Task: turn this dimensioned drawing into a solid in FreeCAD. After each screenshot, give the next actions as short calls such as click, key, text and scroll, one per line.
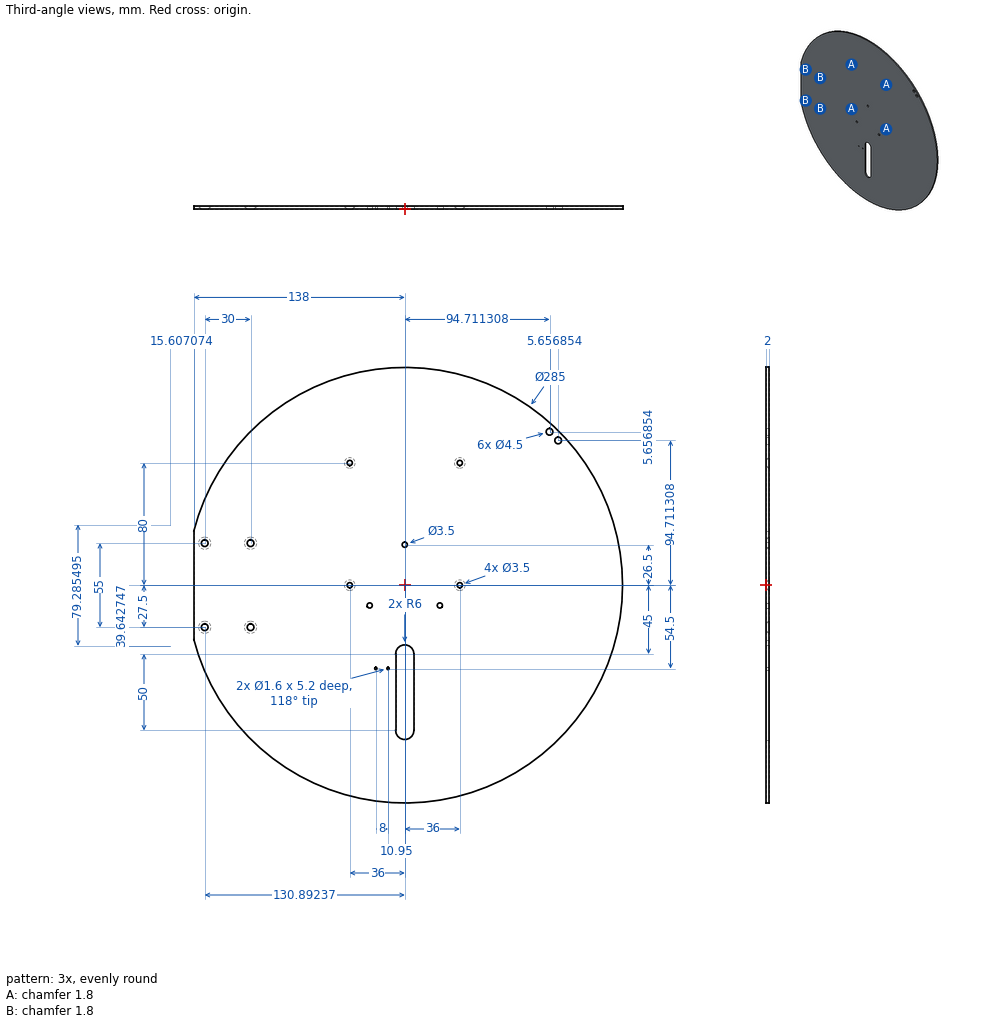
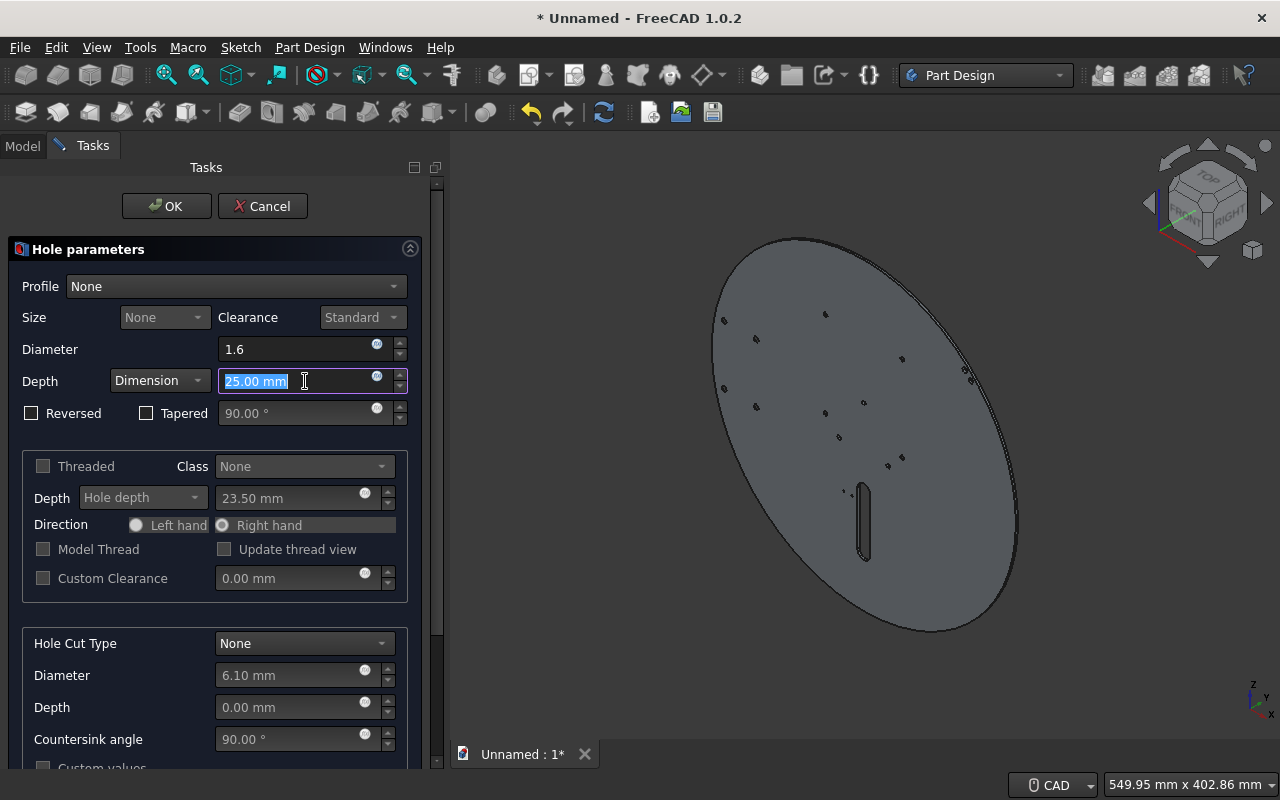
text(5.2)
key(Tab)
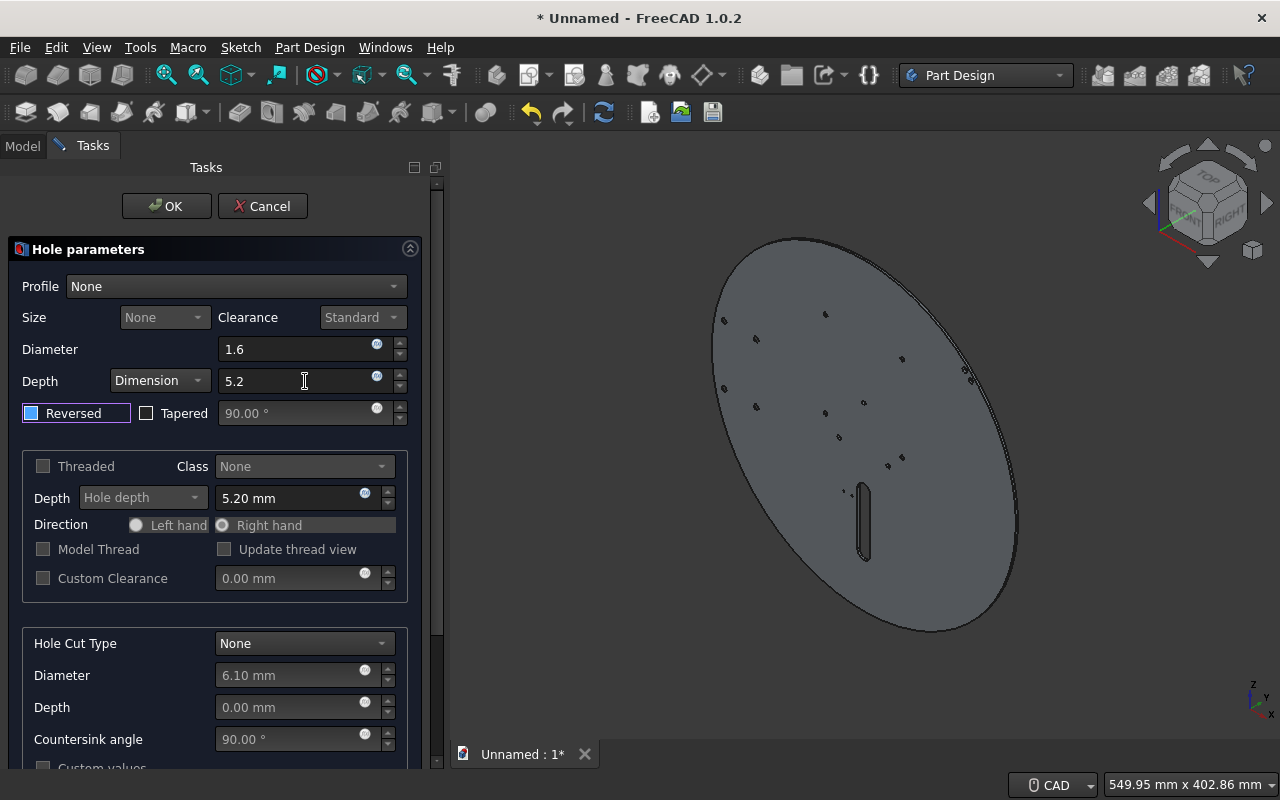
click(167, 206)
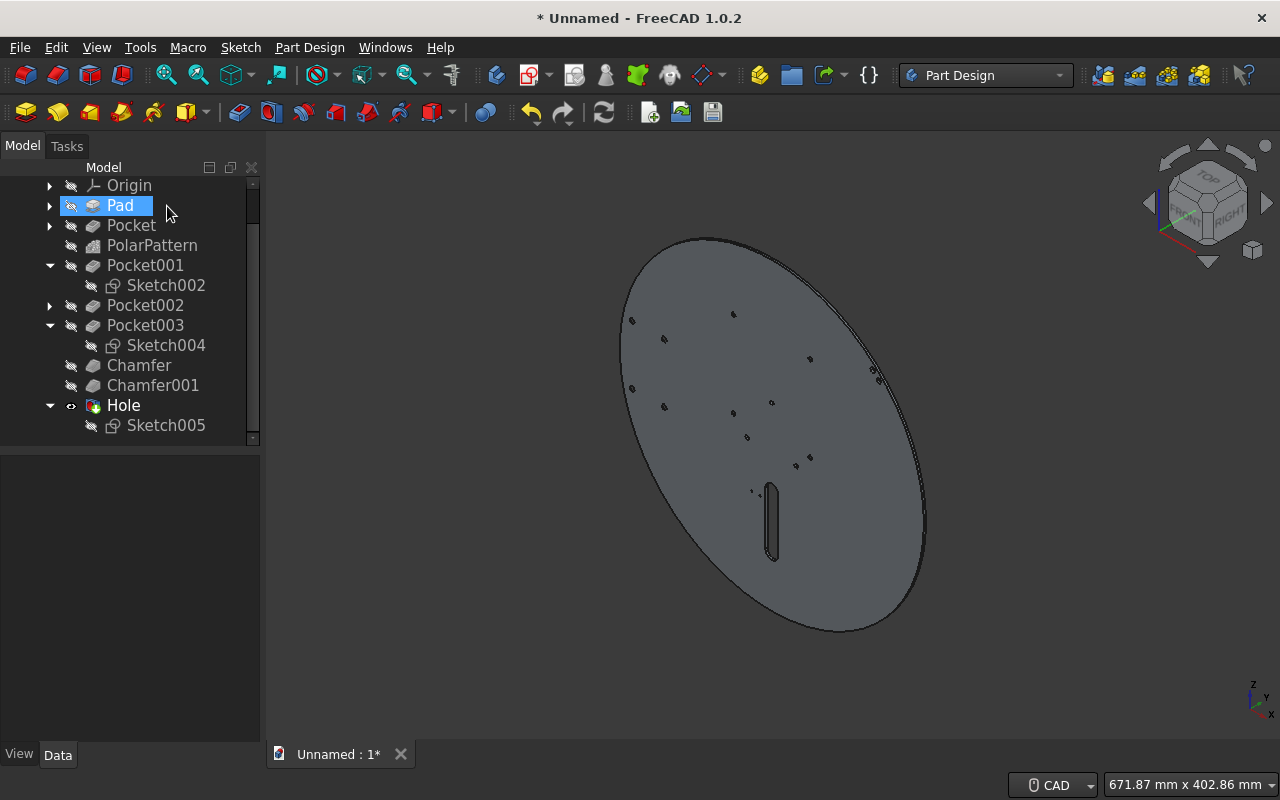
key(4)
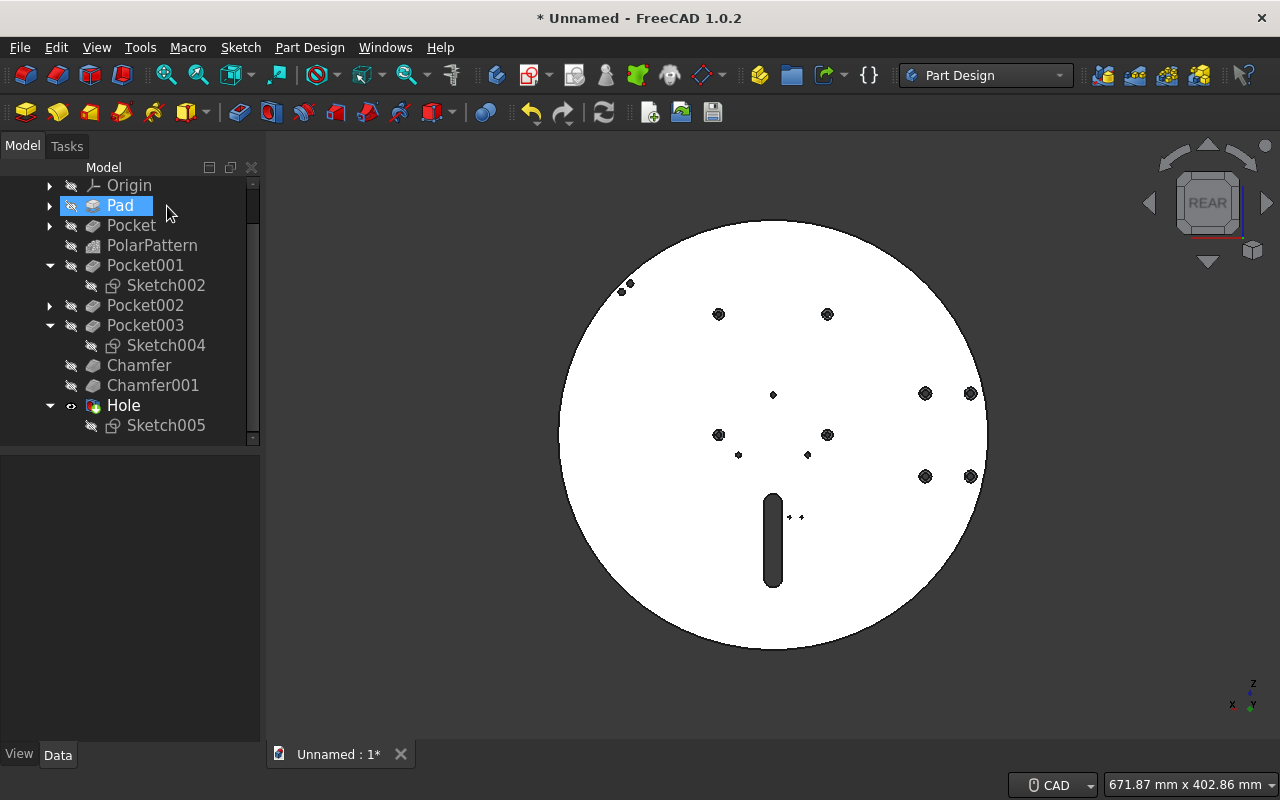
click(650, 495)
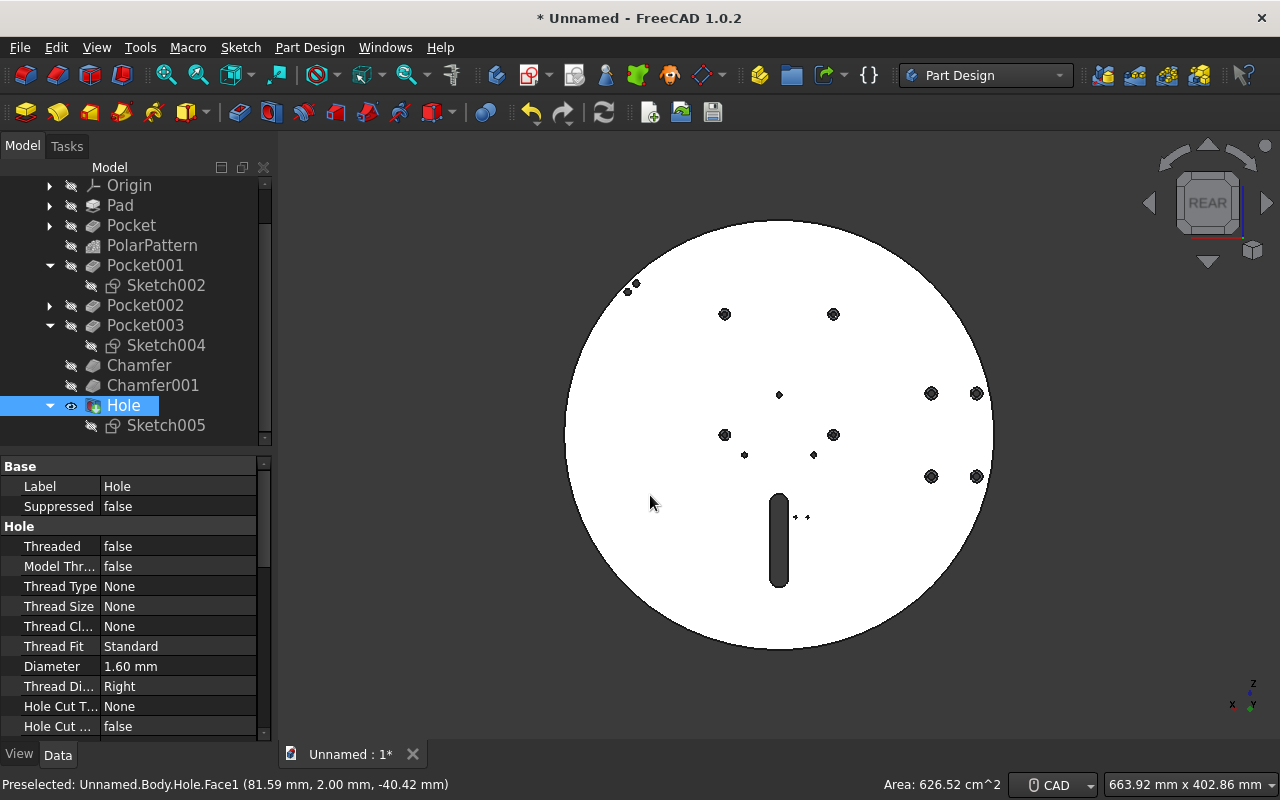
click(530, 76)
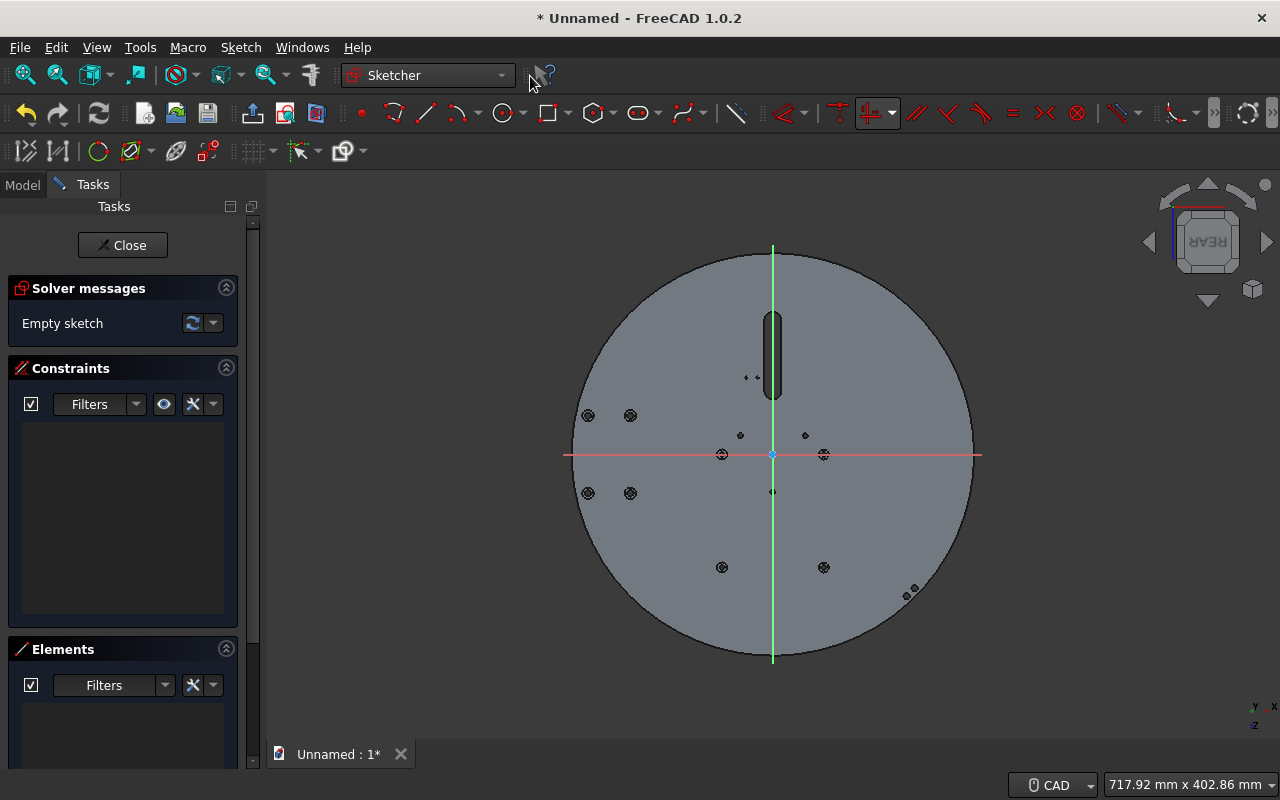
scroll(641, 454, up, 5)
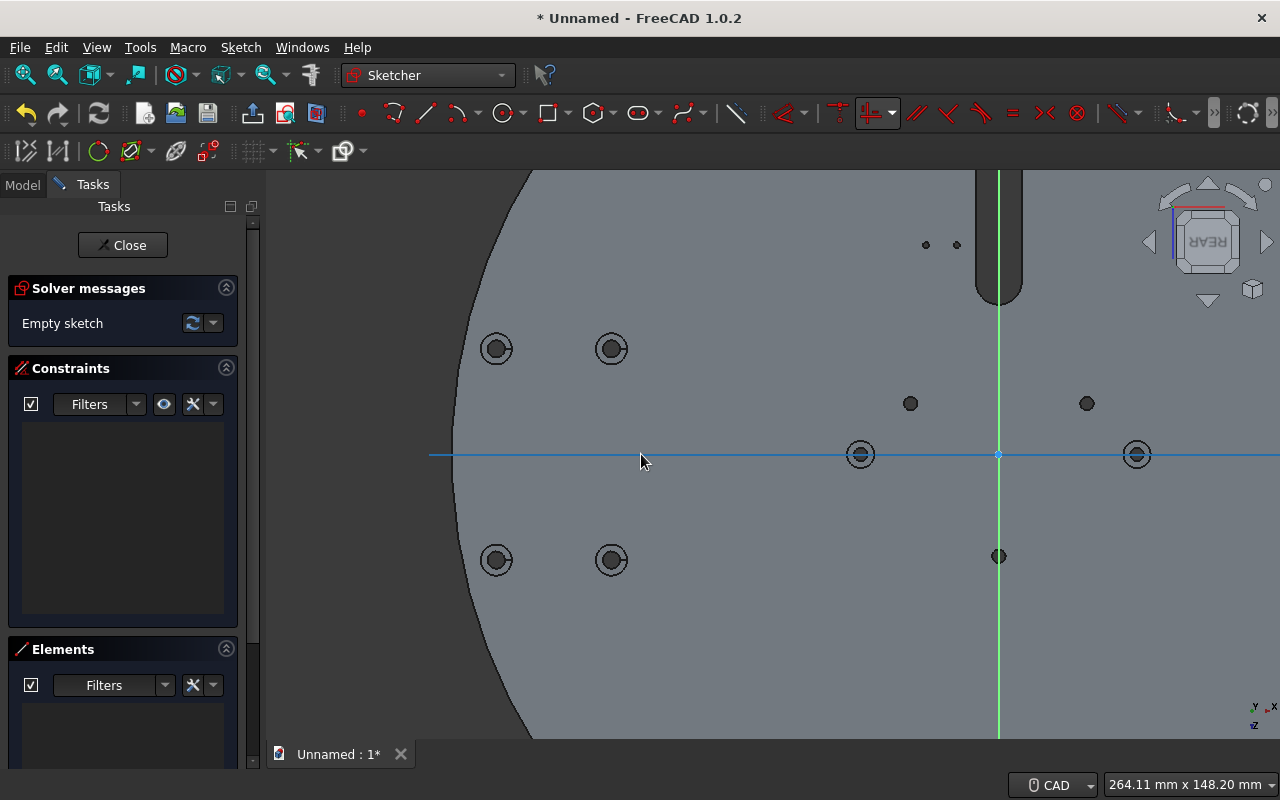
click(548, 114)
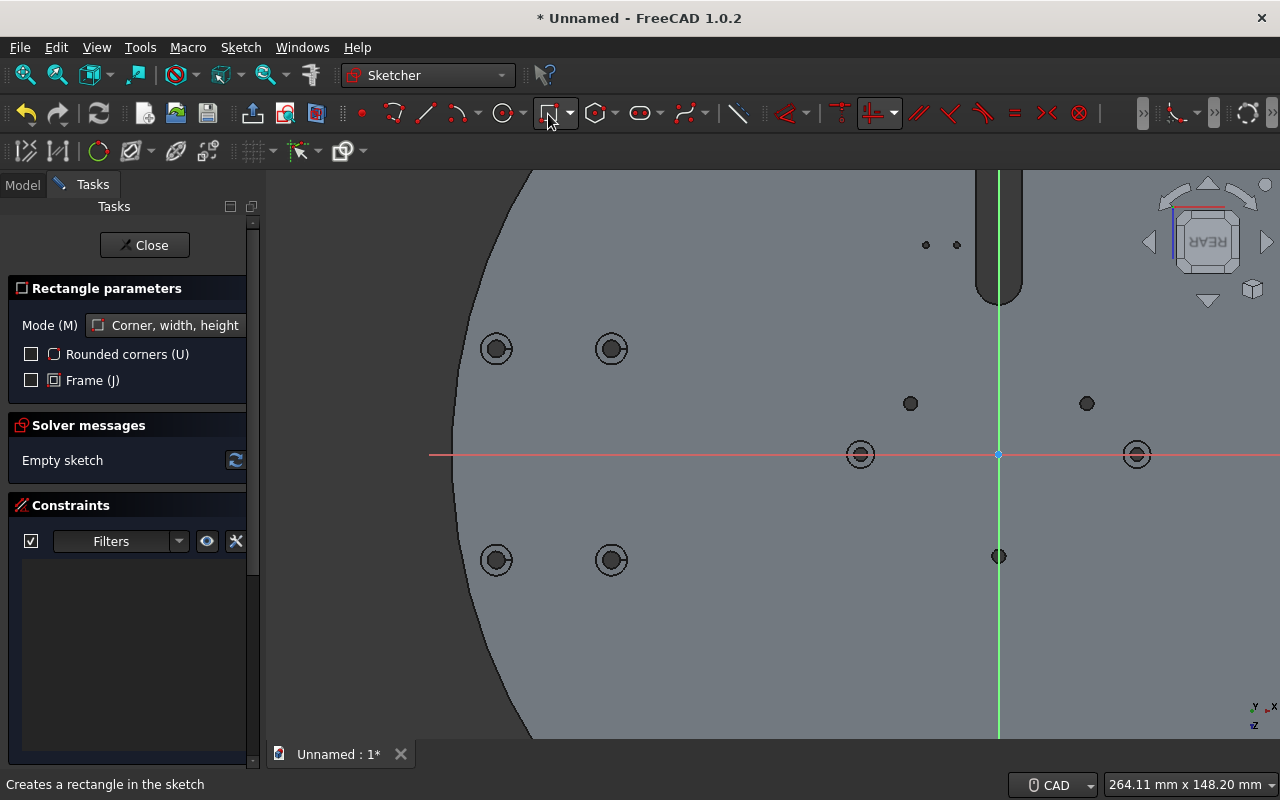
click(409, 302)
click(469, 607)
key(Escape)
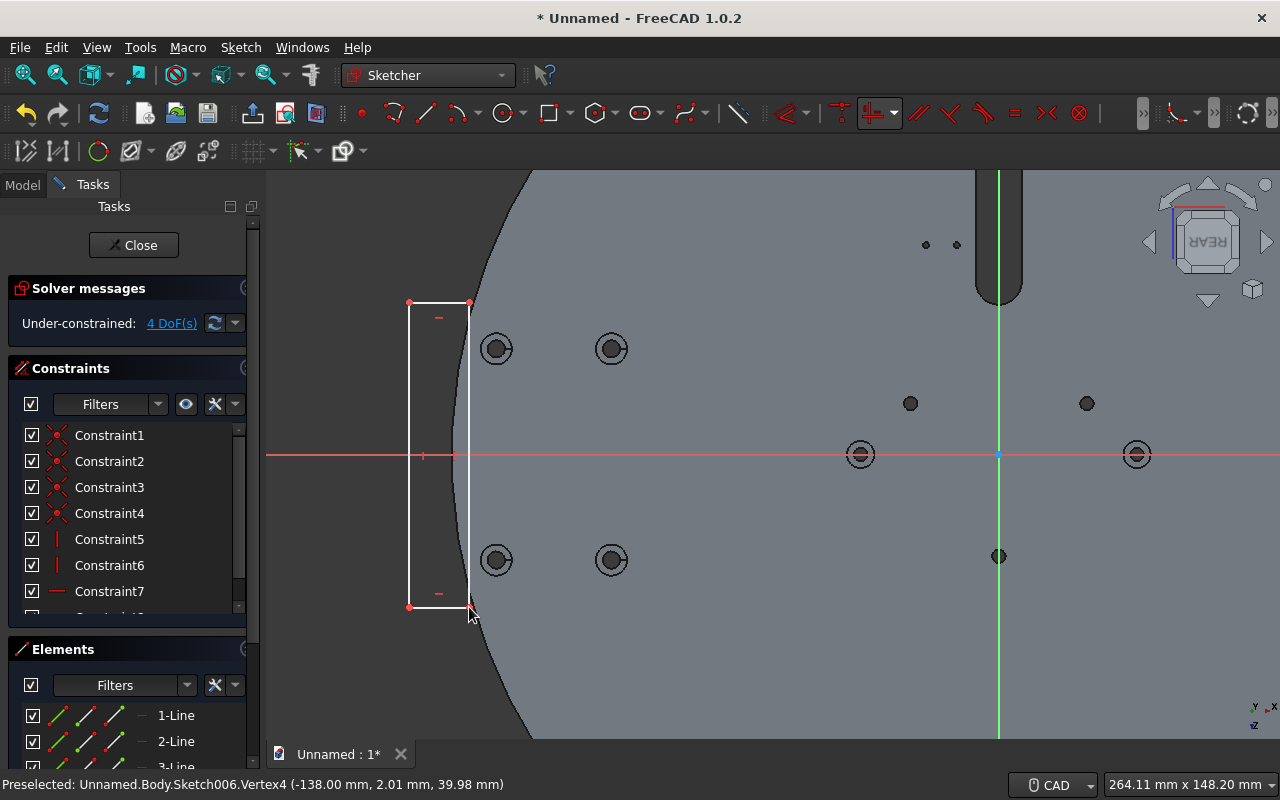
click(786, 114)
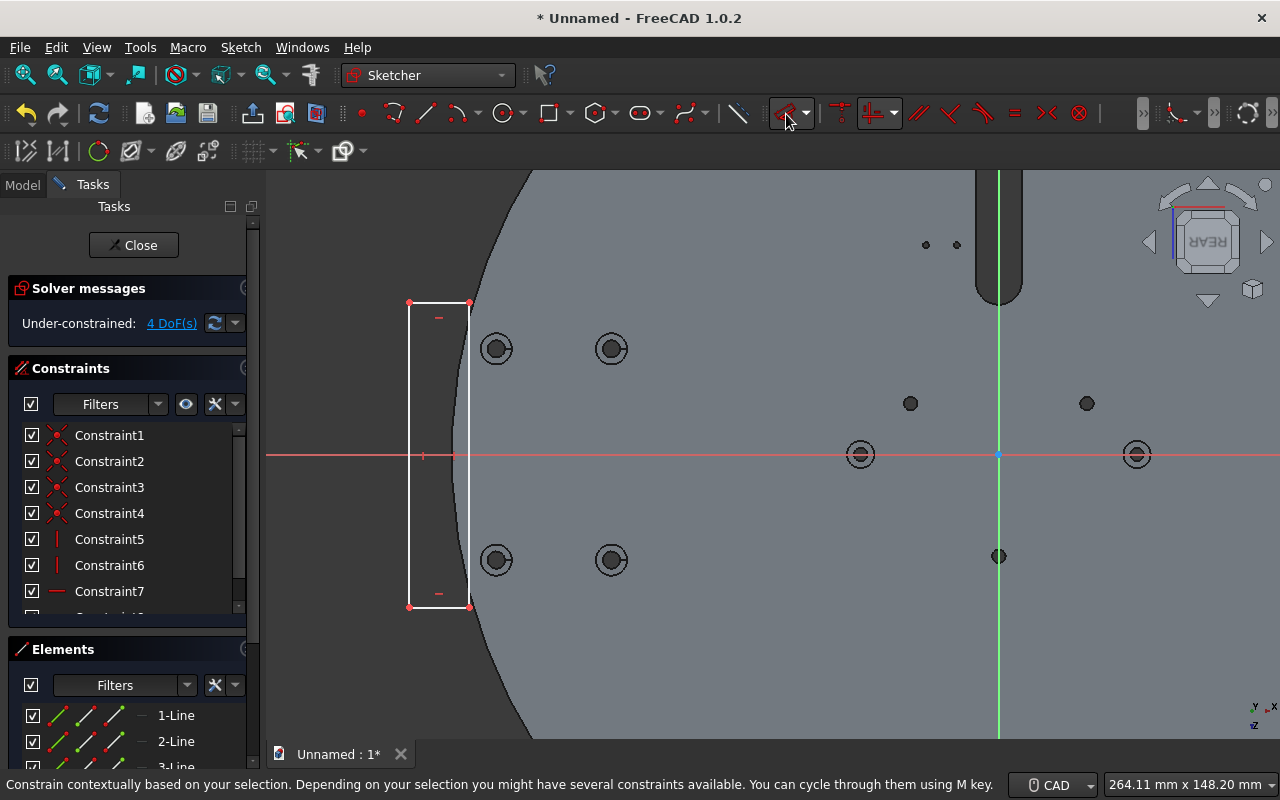
click(469, 608)
click(734, 642)